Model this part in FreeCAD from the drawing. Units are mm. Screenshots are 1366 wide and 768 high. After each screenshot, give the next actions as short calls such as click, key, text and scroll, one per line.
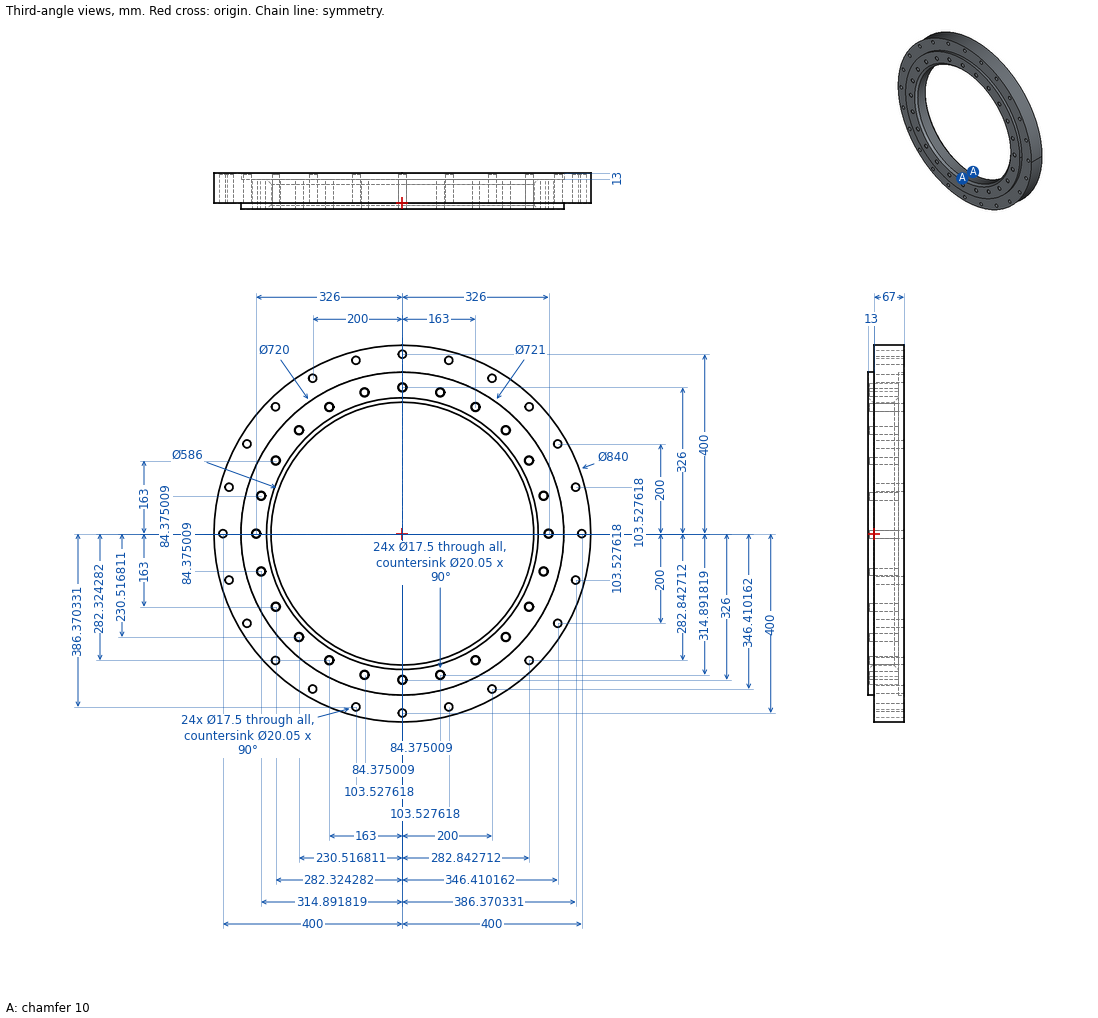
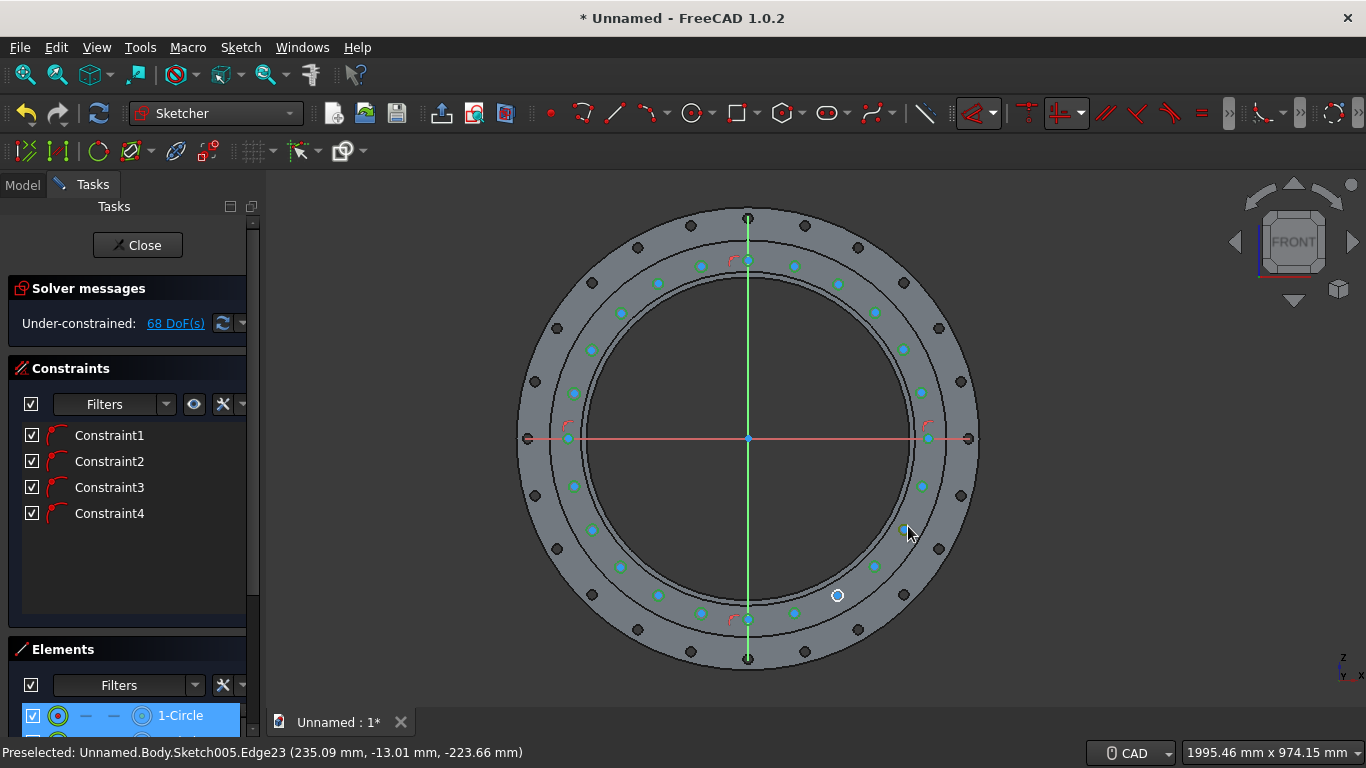
scroll(842, 592, up, 5)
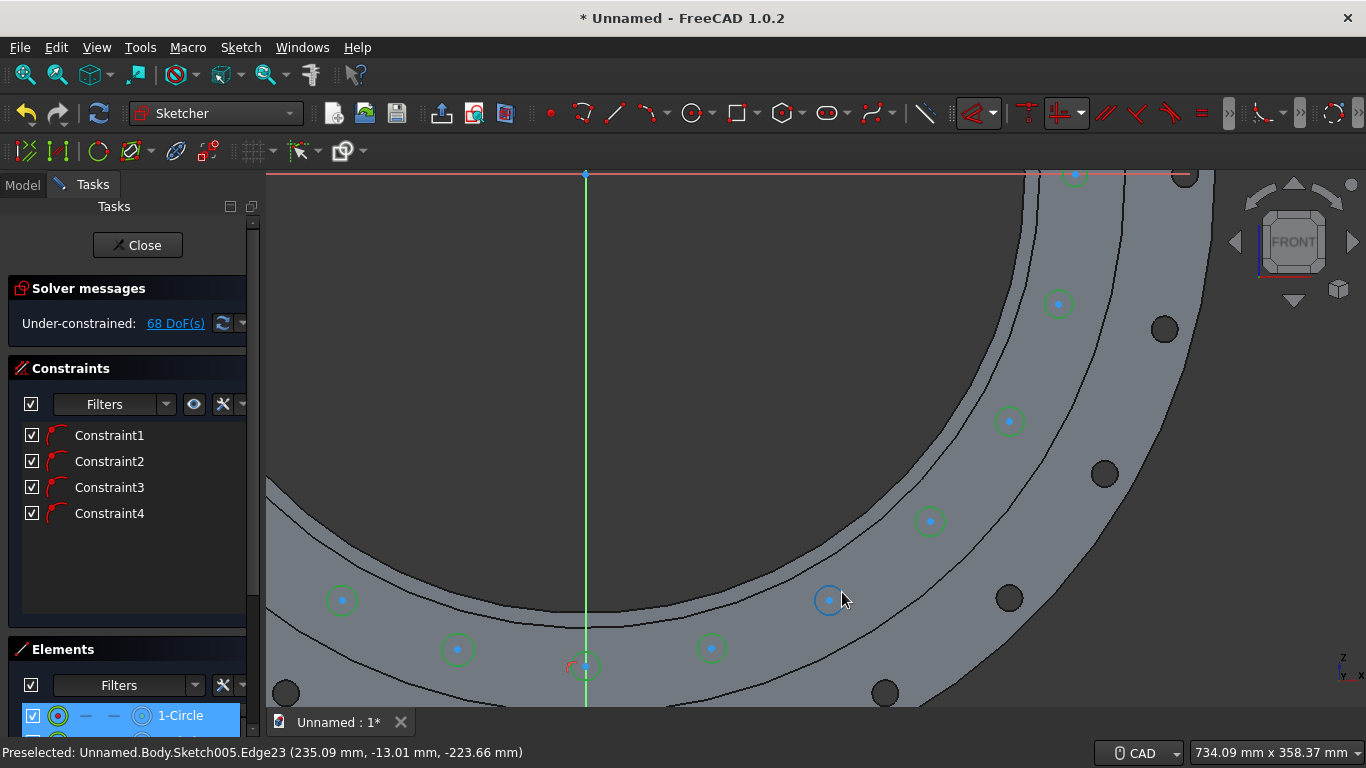
click(840, 590)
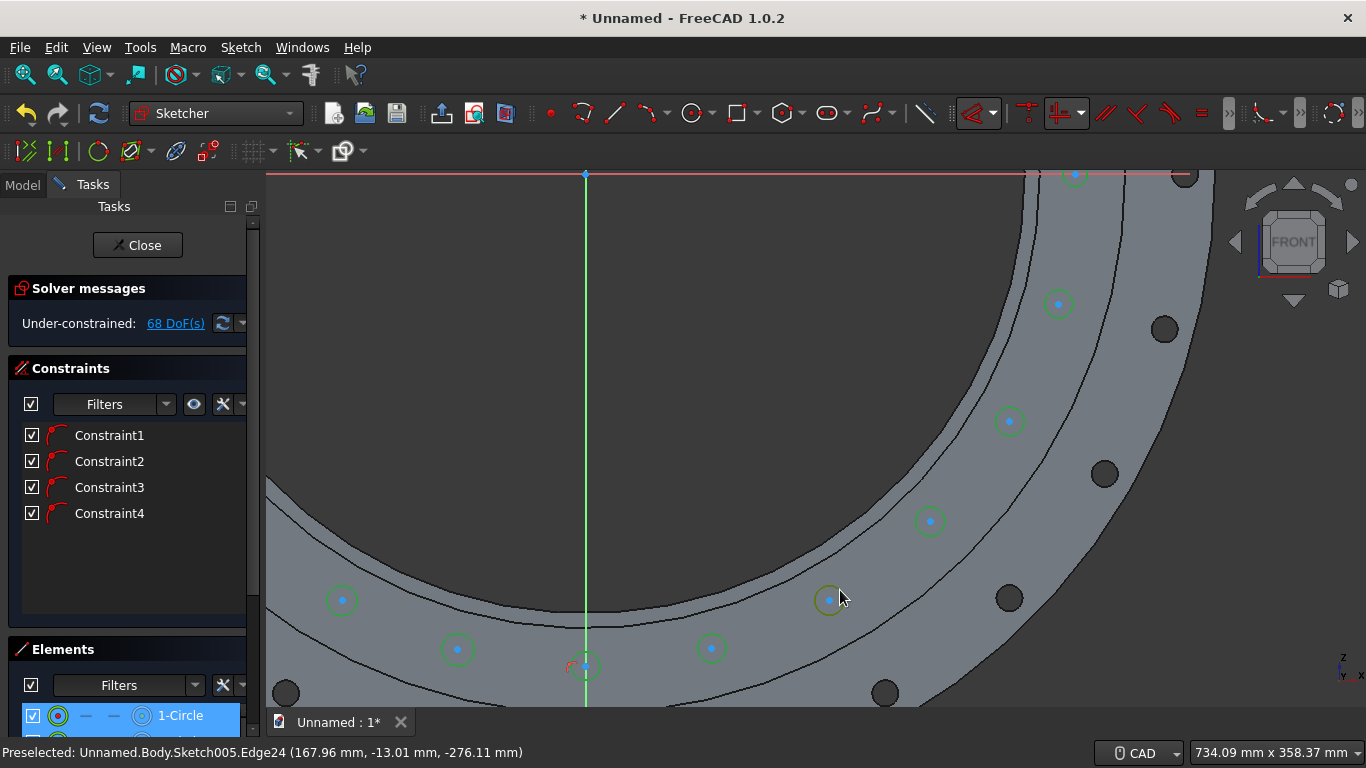
key(e)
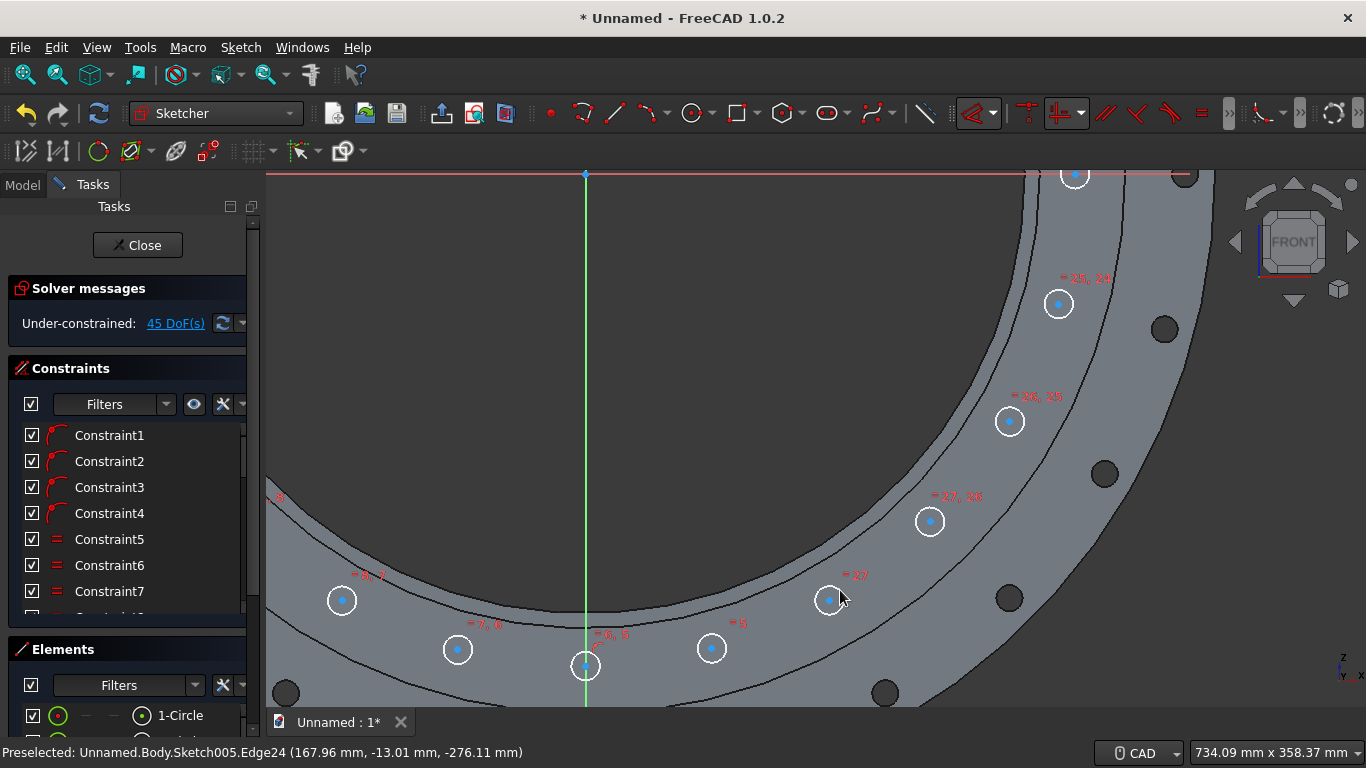
click(712, 648)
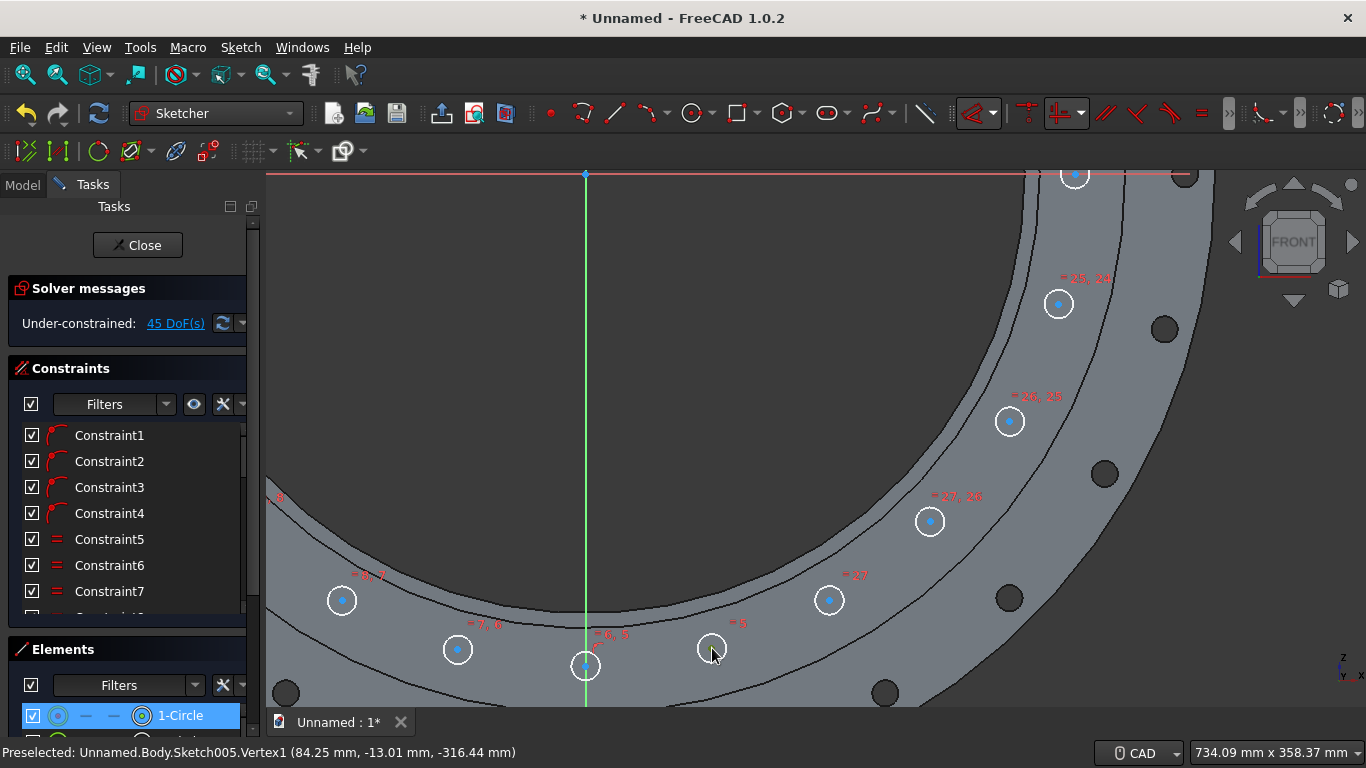
click(458, 650)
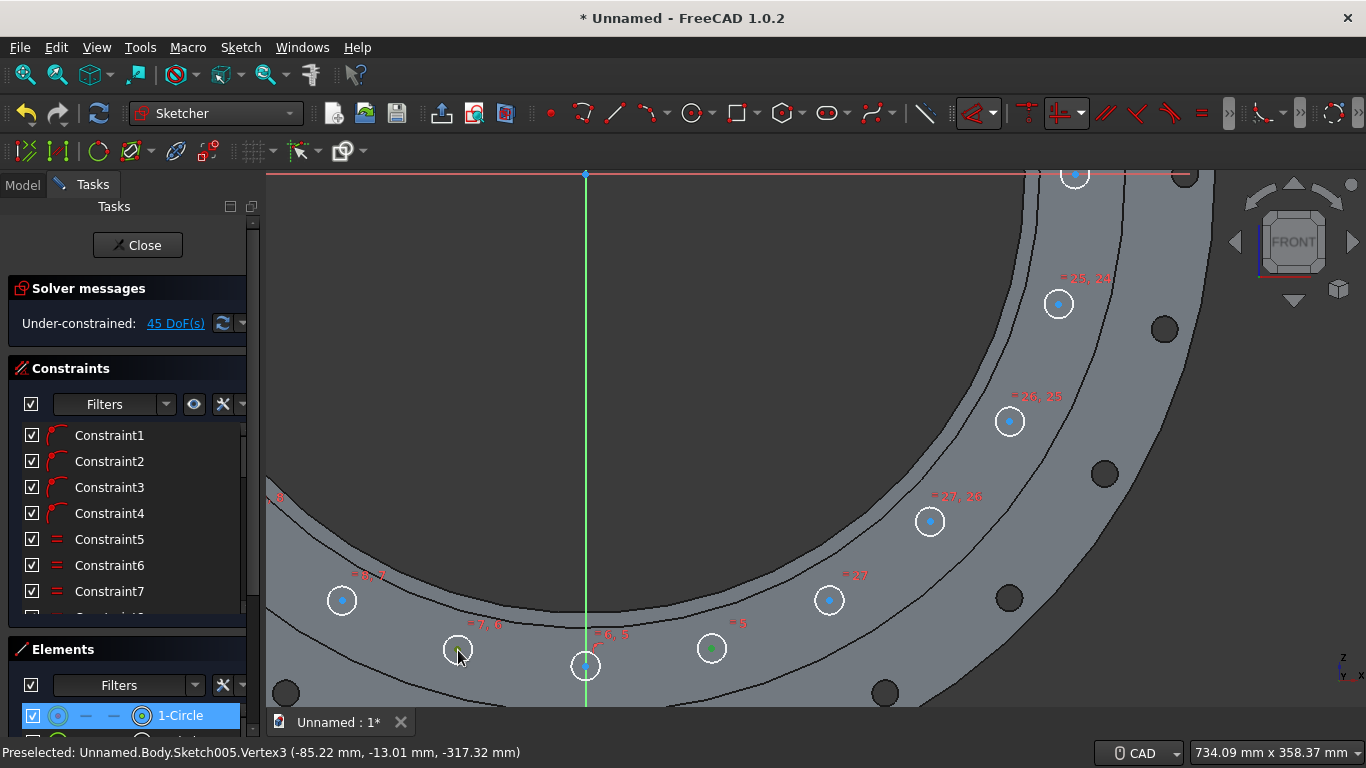
key(h)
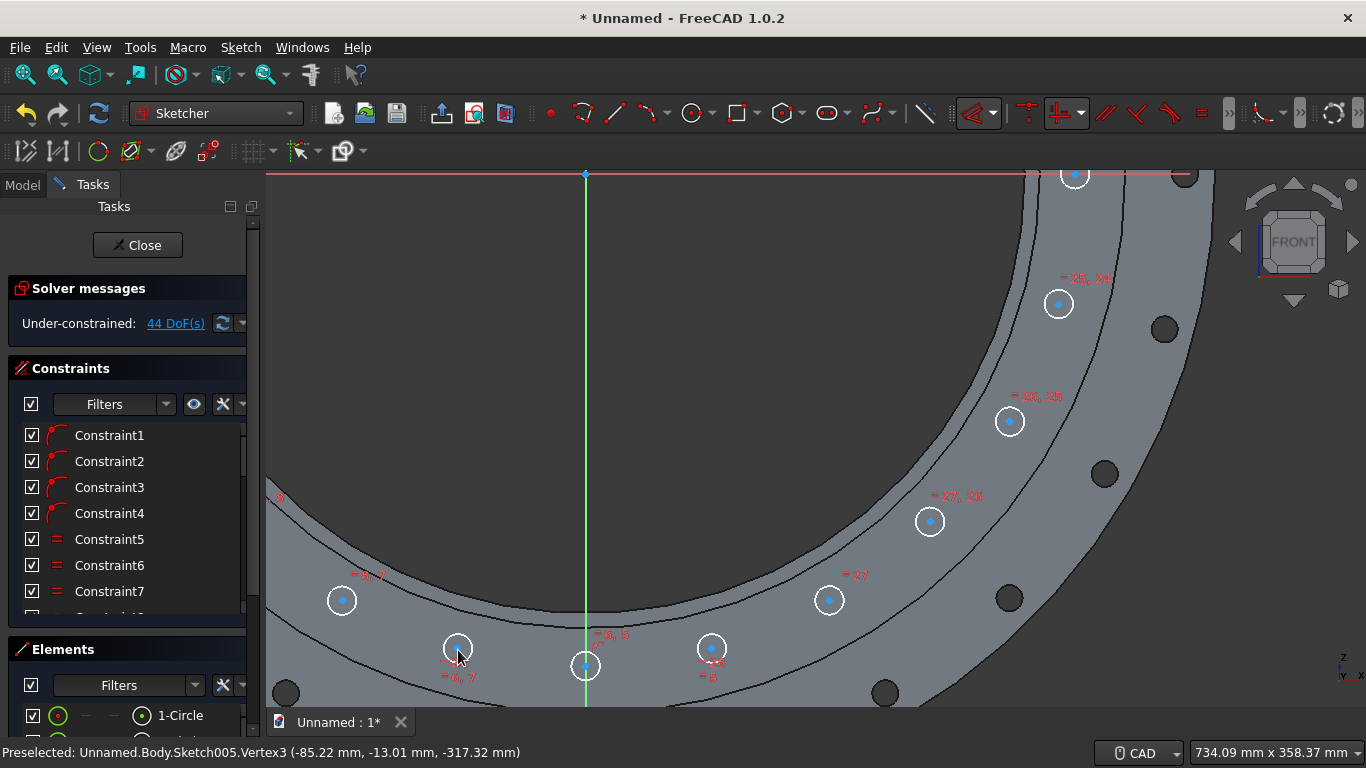
scroll(842, 592, down, 5)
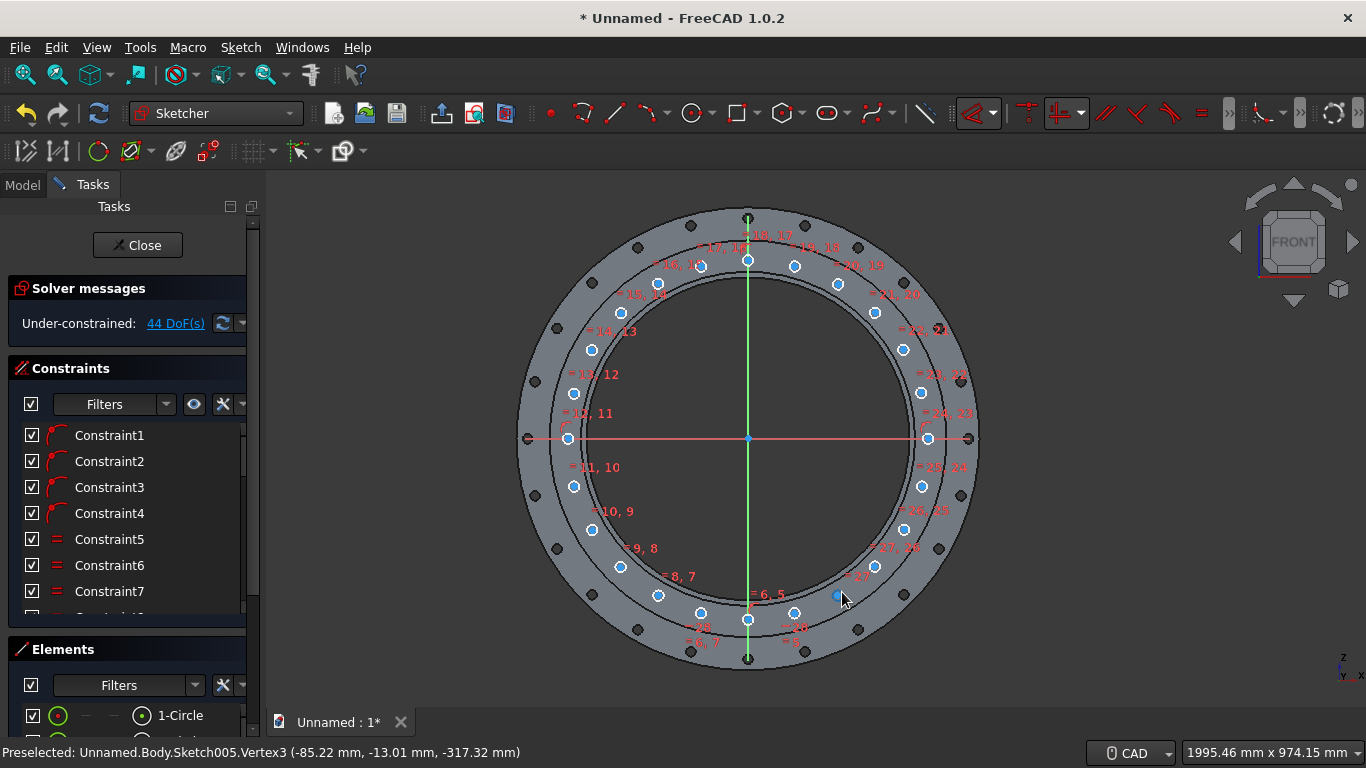
click(574, 487)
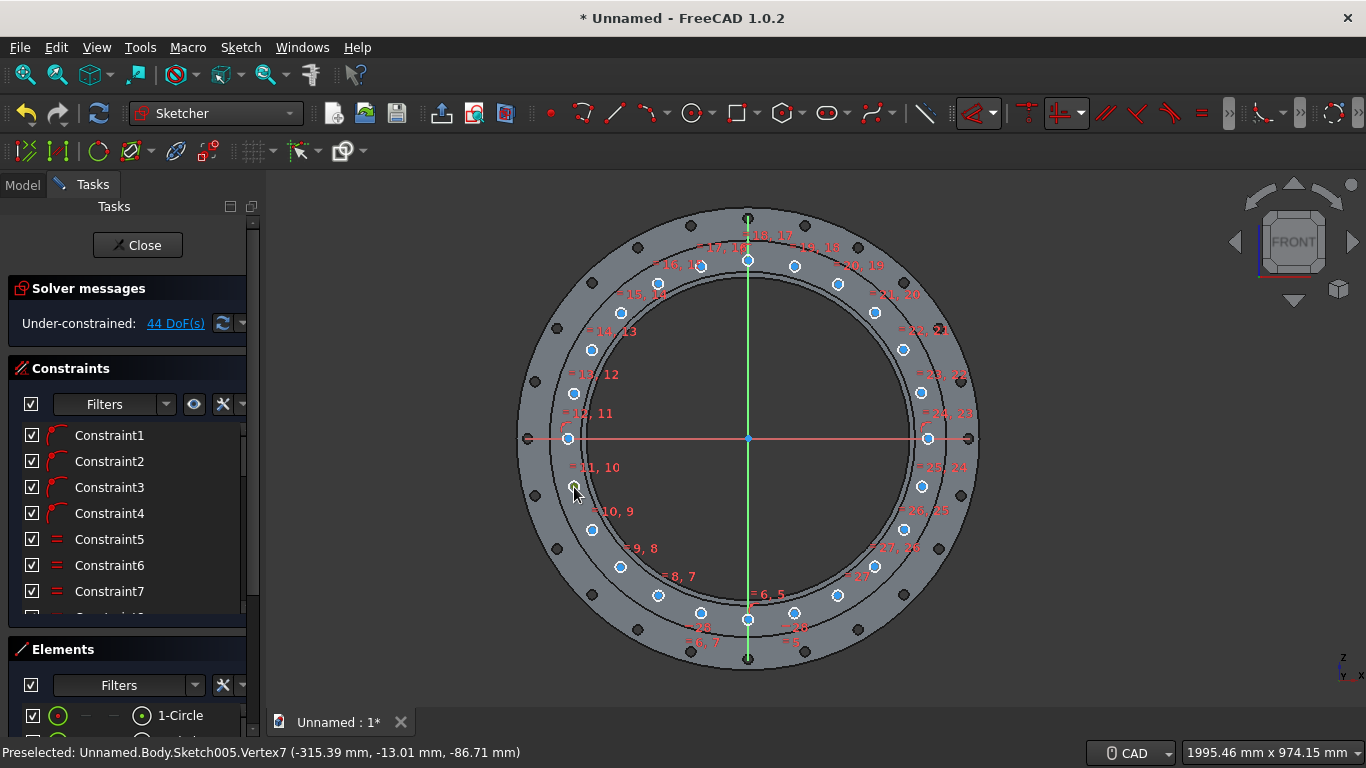
click(574, 394)